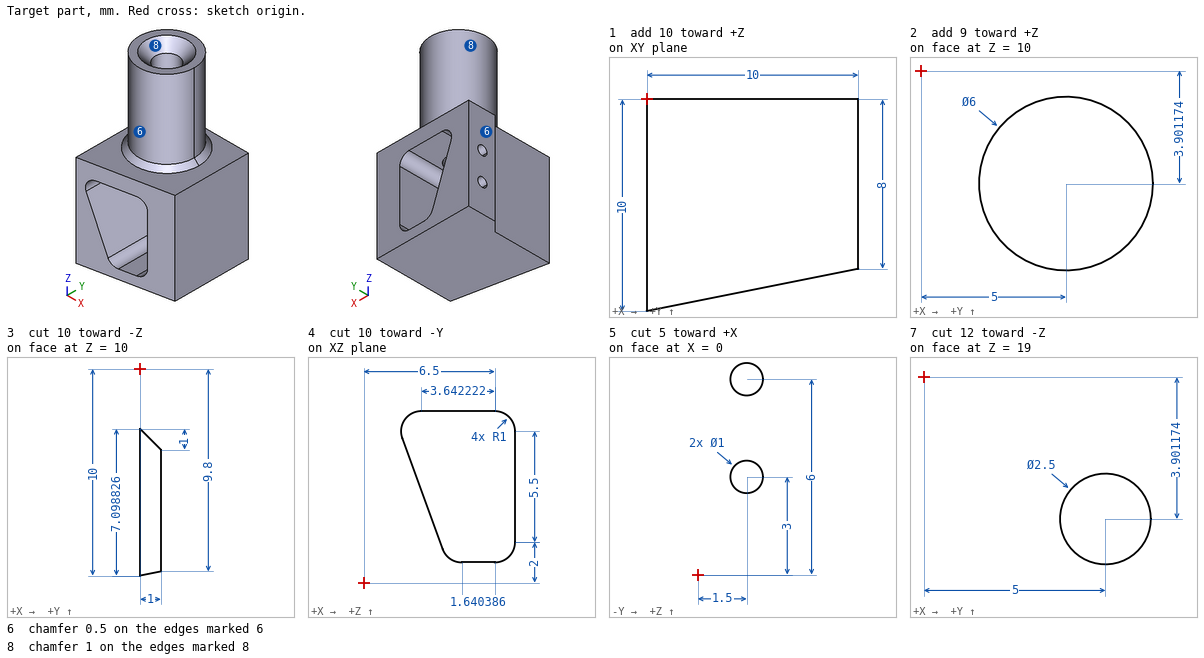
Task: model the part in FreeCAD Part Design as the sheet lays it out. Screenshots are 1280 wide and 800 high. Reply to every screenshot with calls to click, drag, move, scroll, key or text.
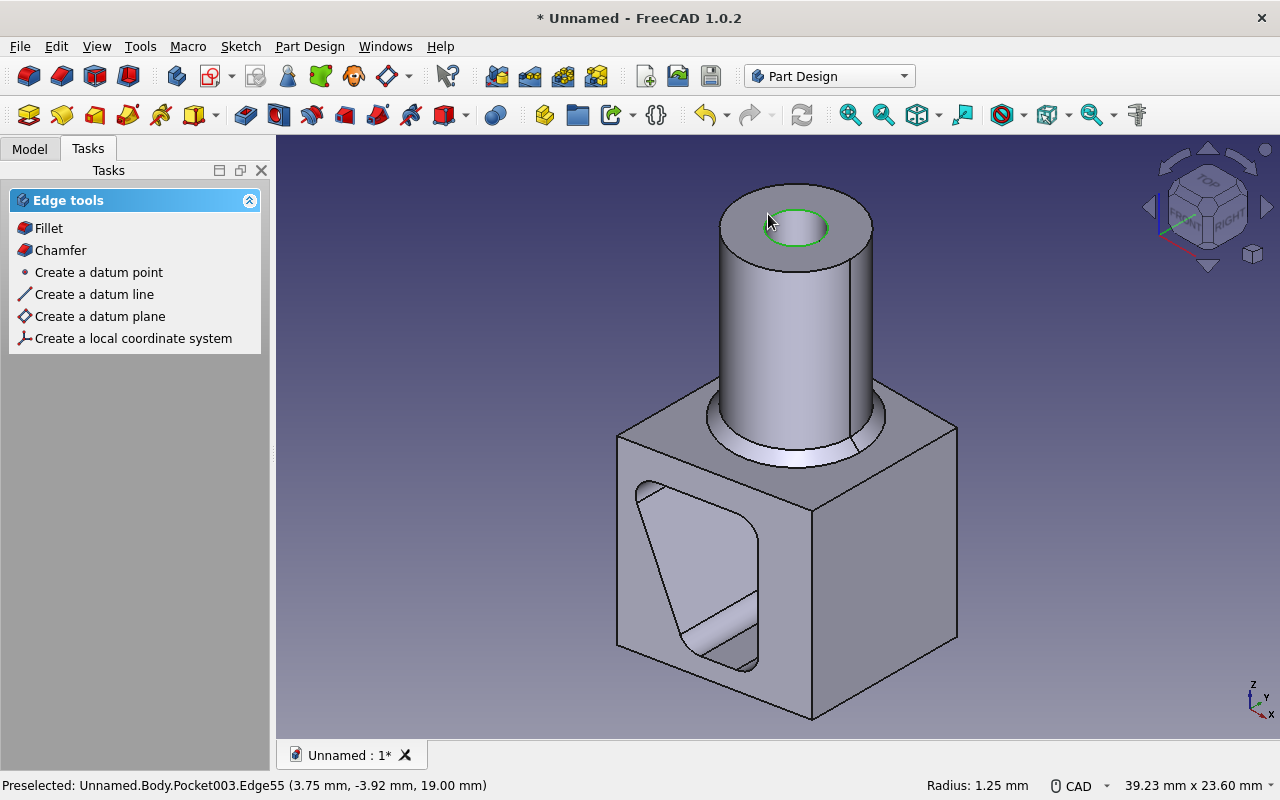
click(62, 76)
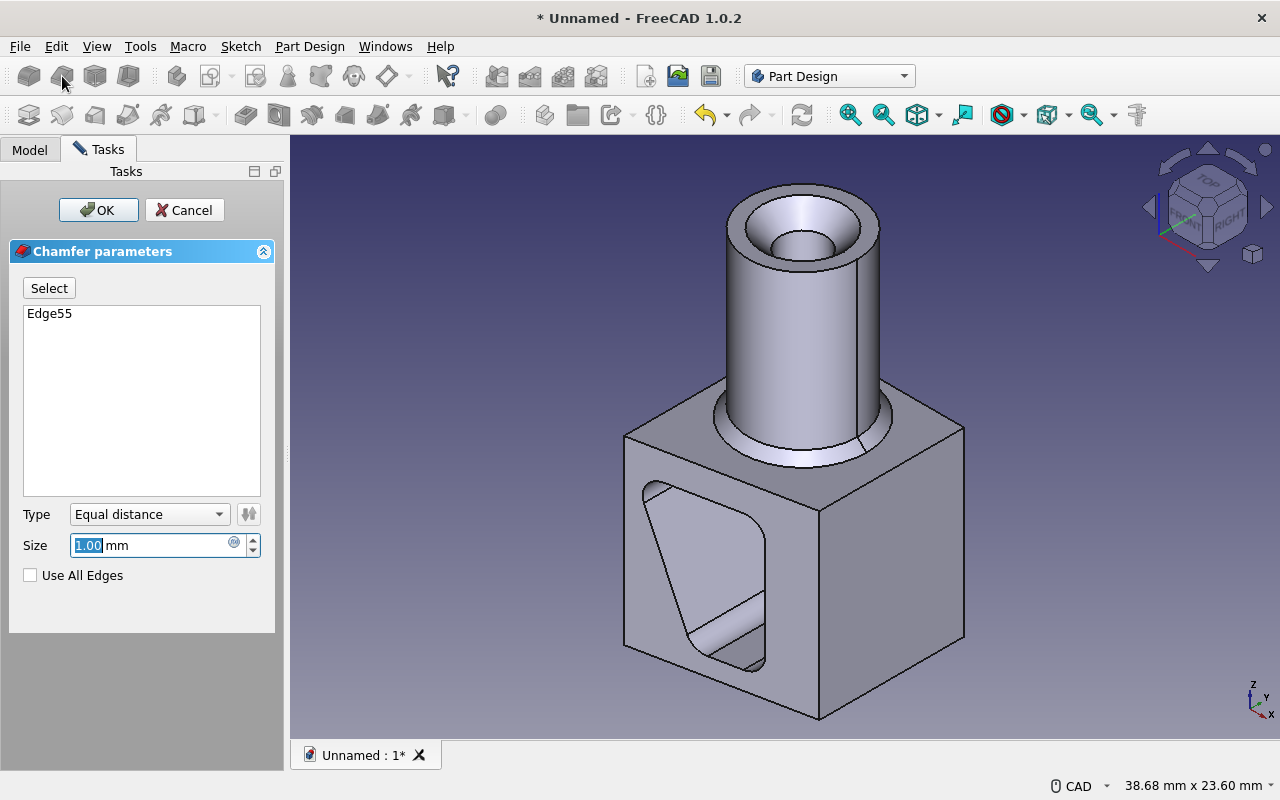
text(1)
key(Tab)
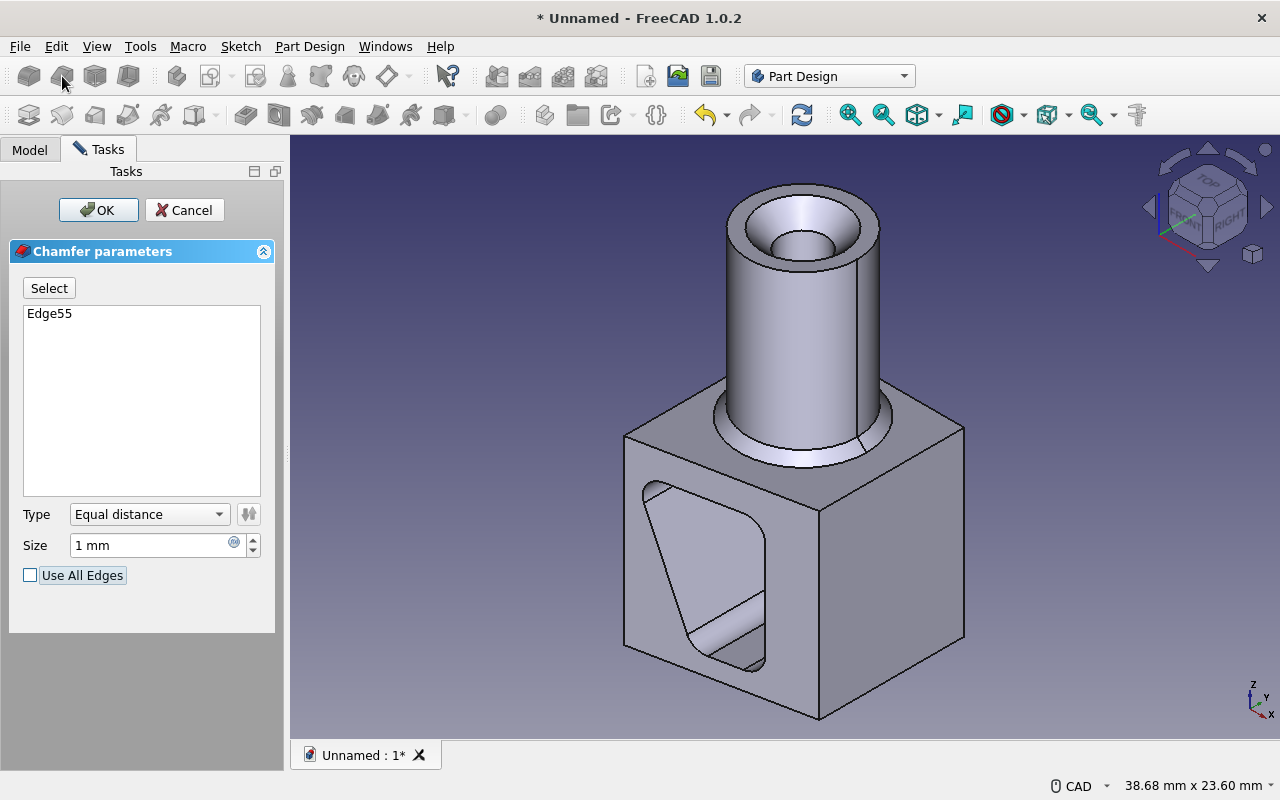
click(99, 210)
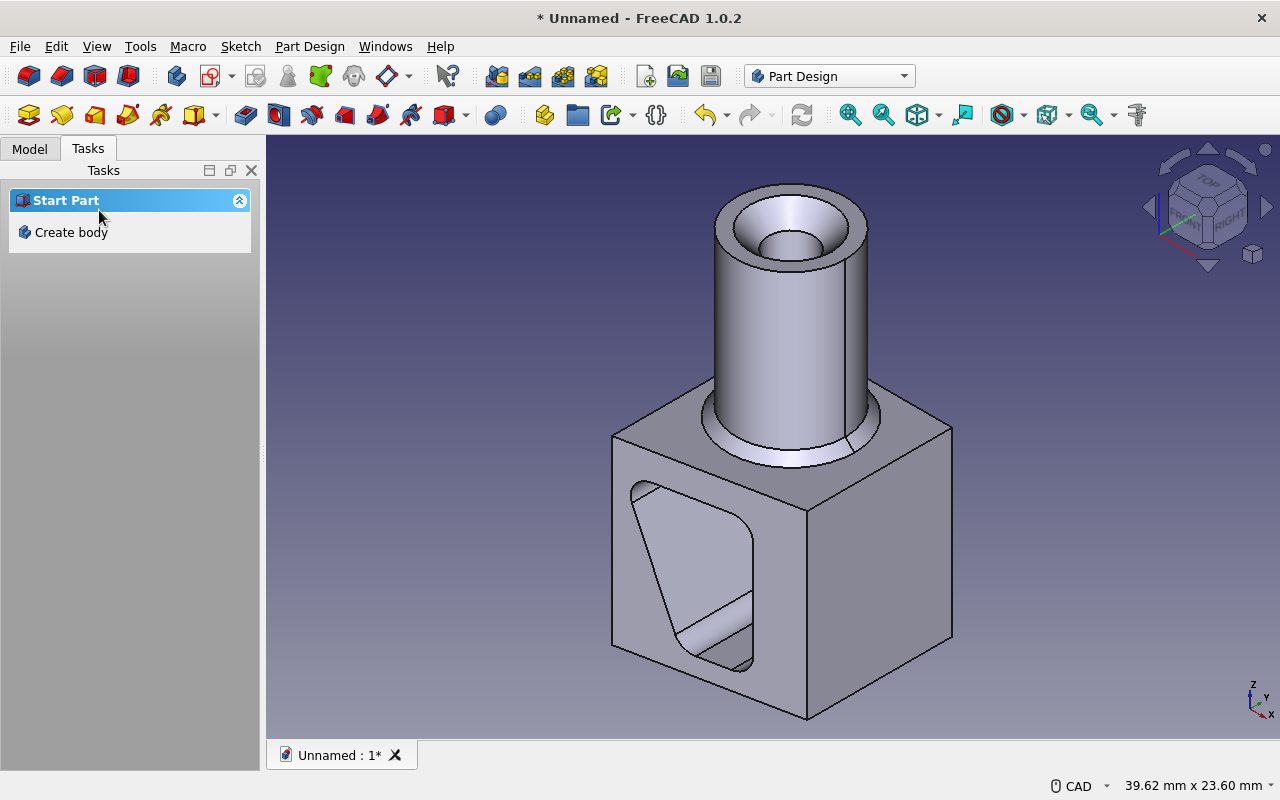
key(v)
key(f)